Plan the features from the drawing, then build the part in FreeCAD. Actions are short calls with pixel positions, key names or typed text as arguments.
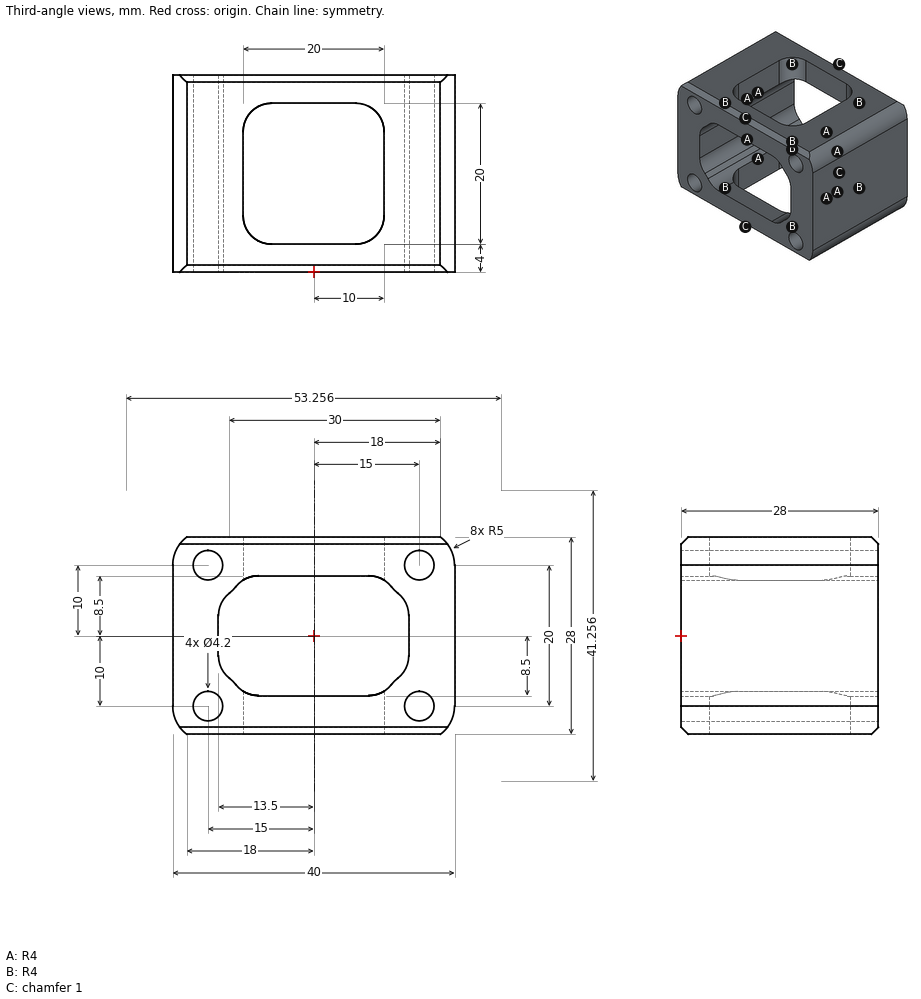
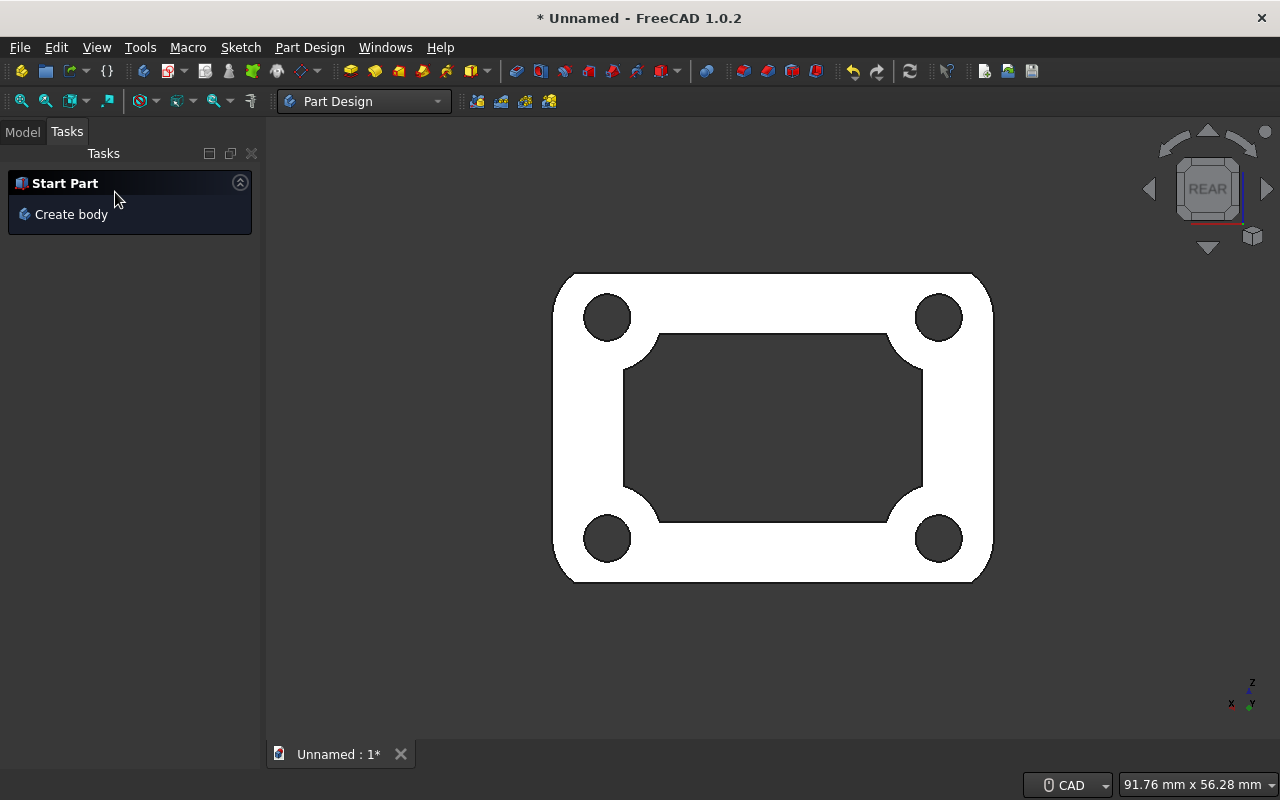
key(0)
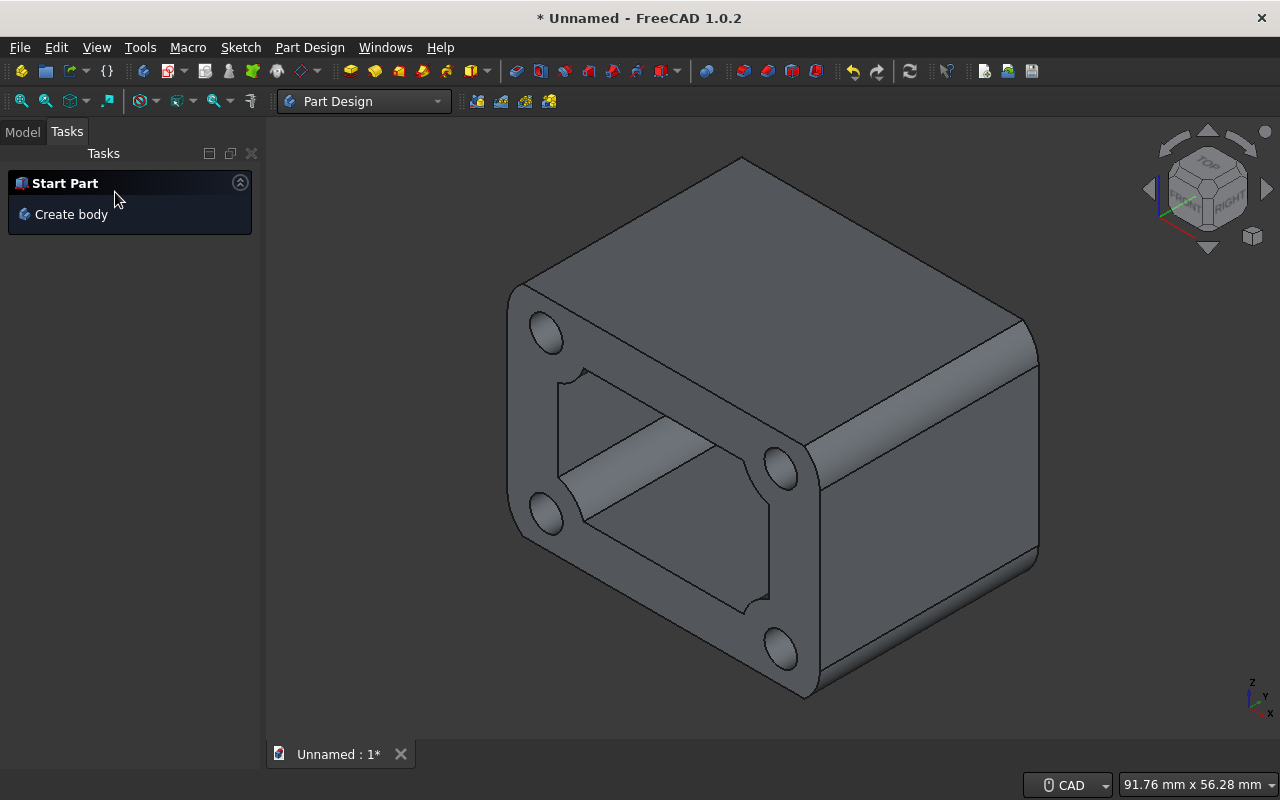
key(2)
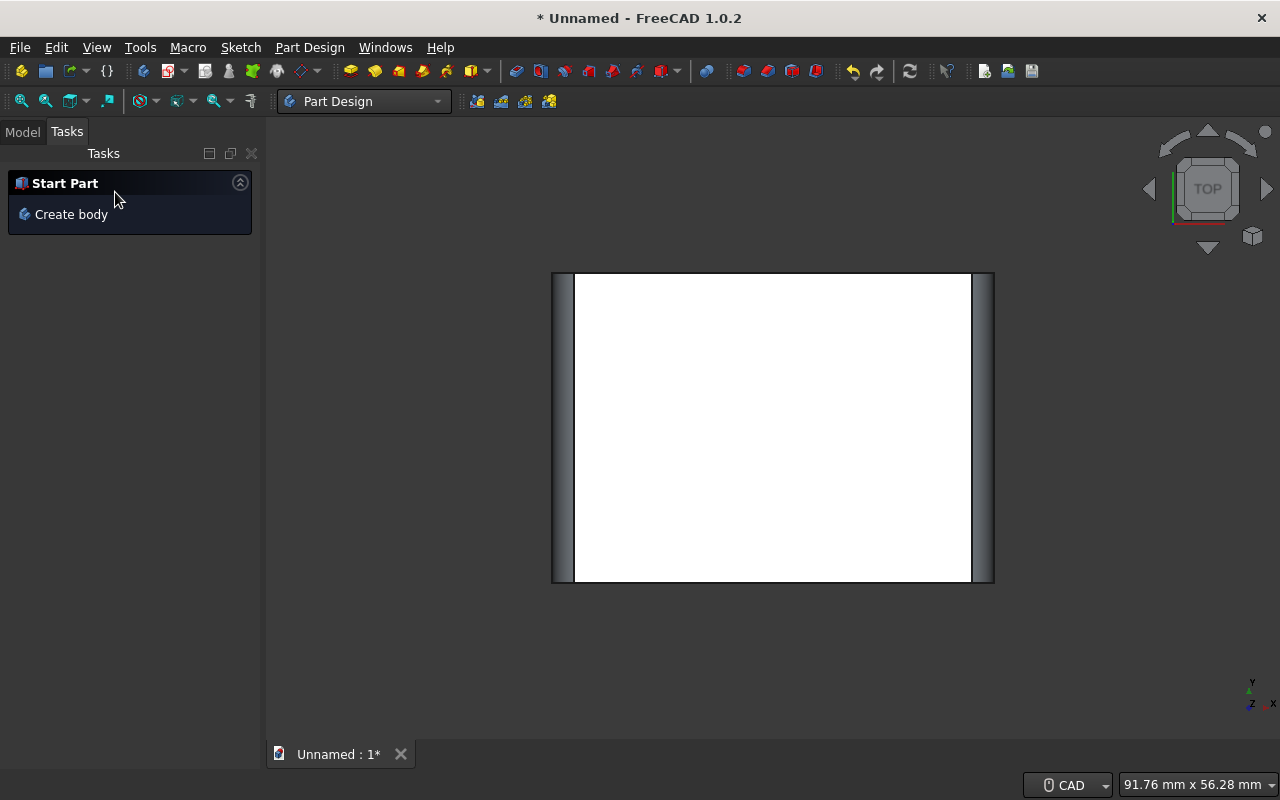
key(1)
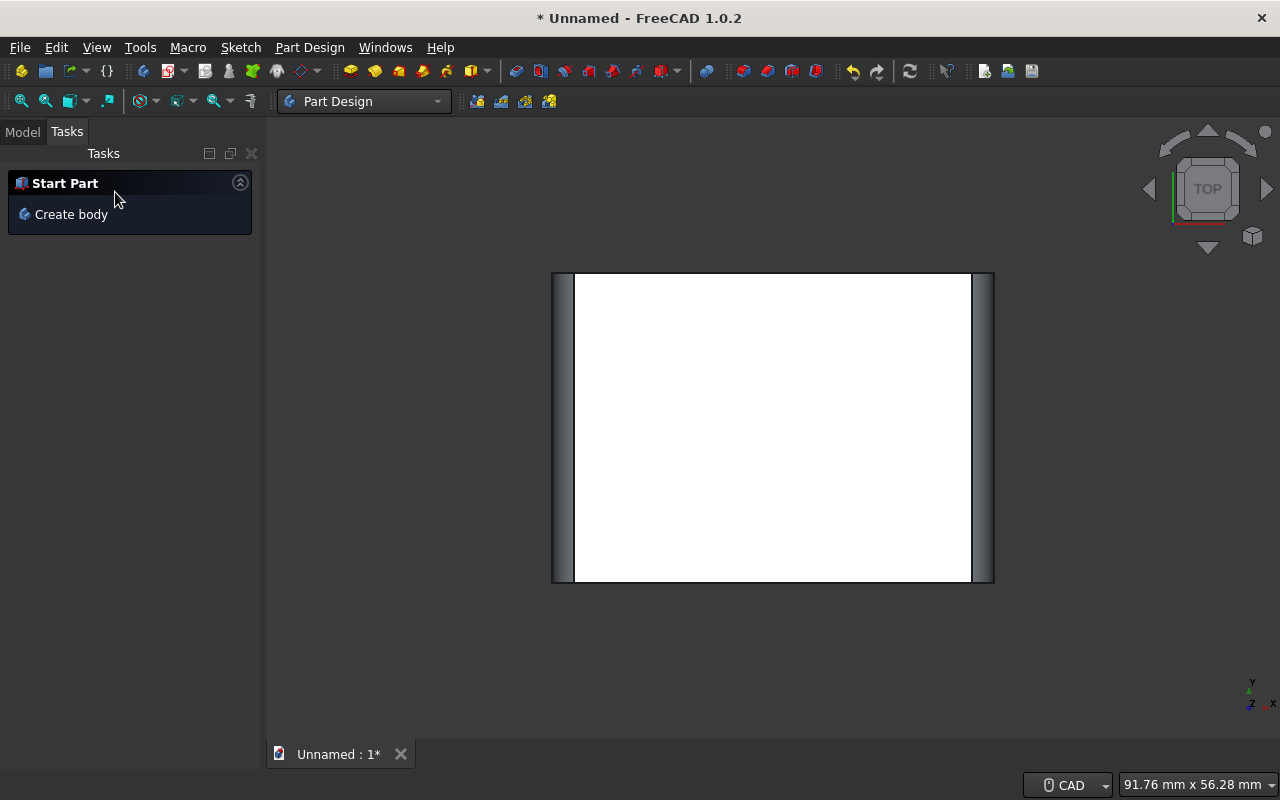
key(3)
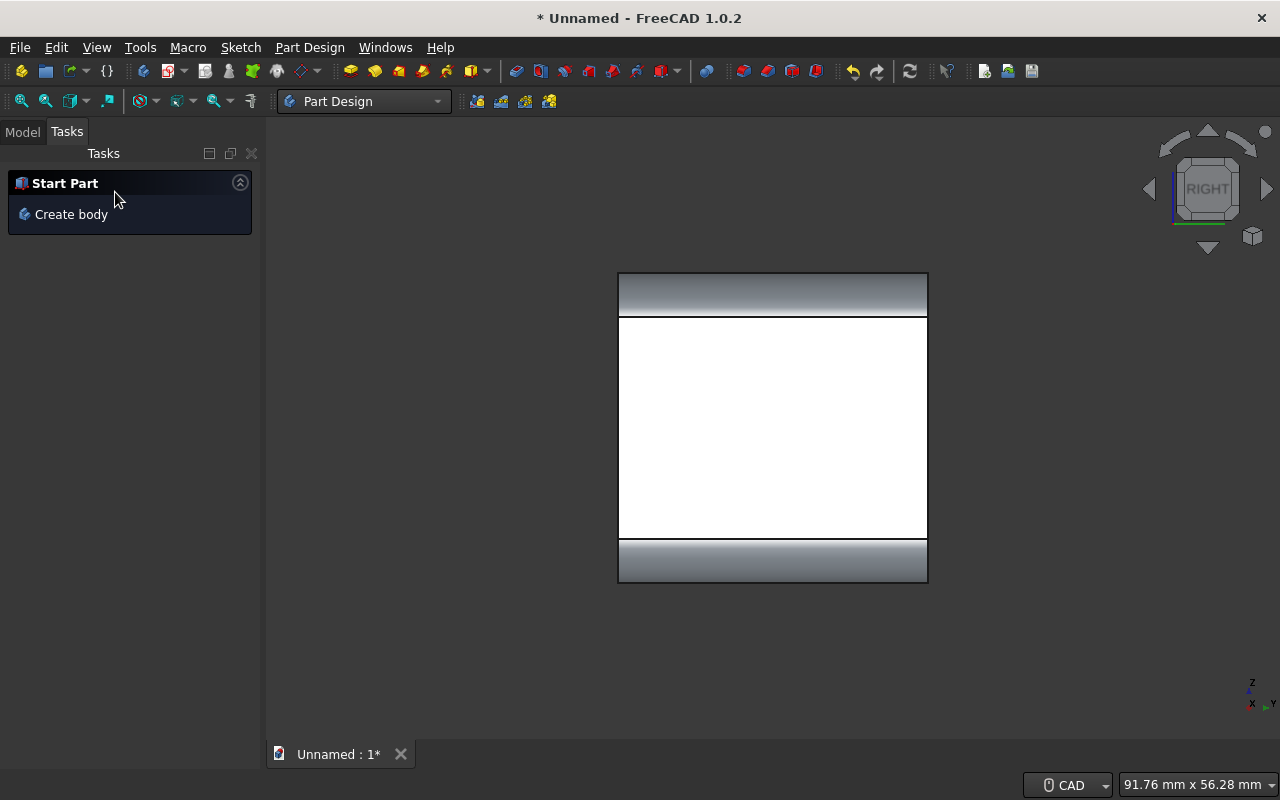
key(5)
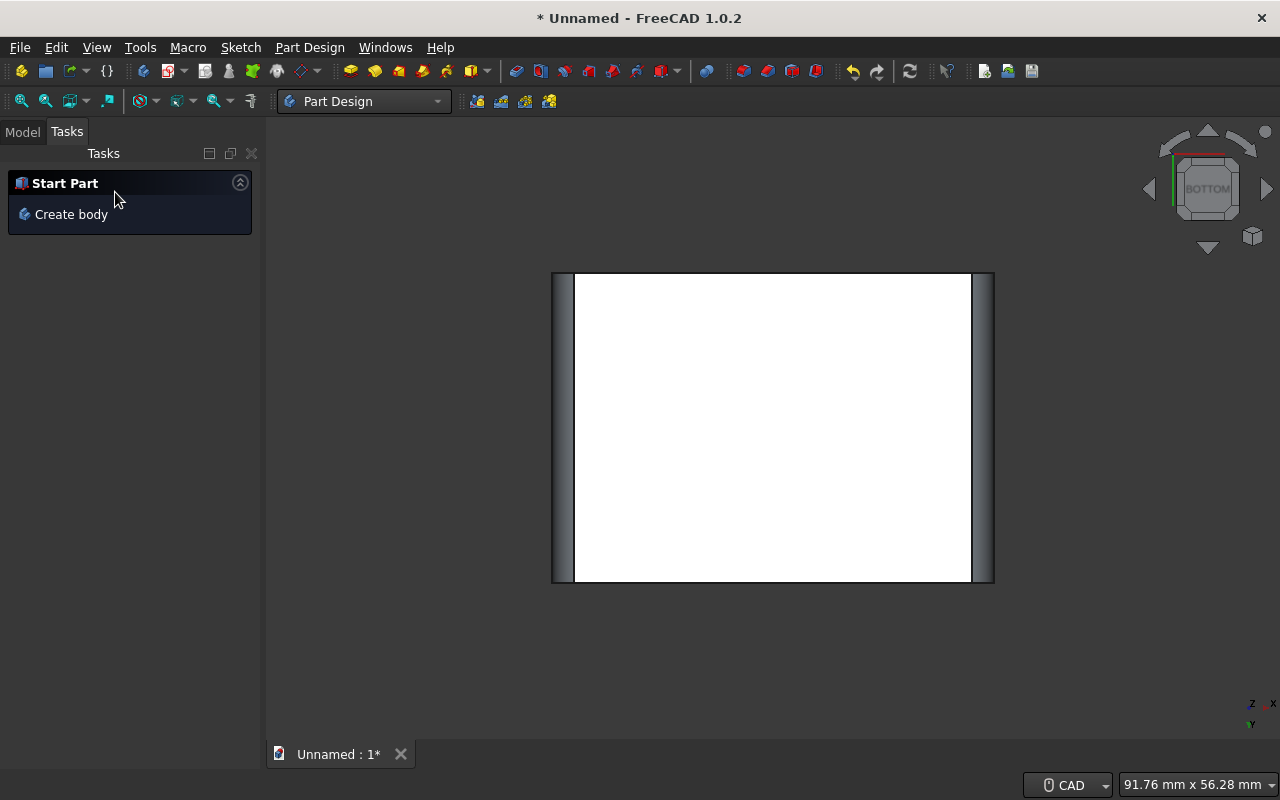
key(4)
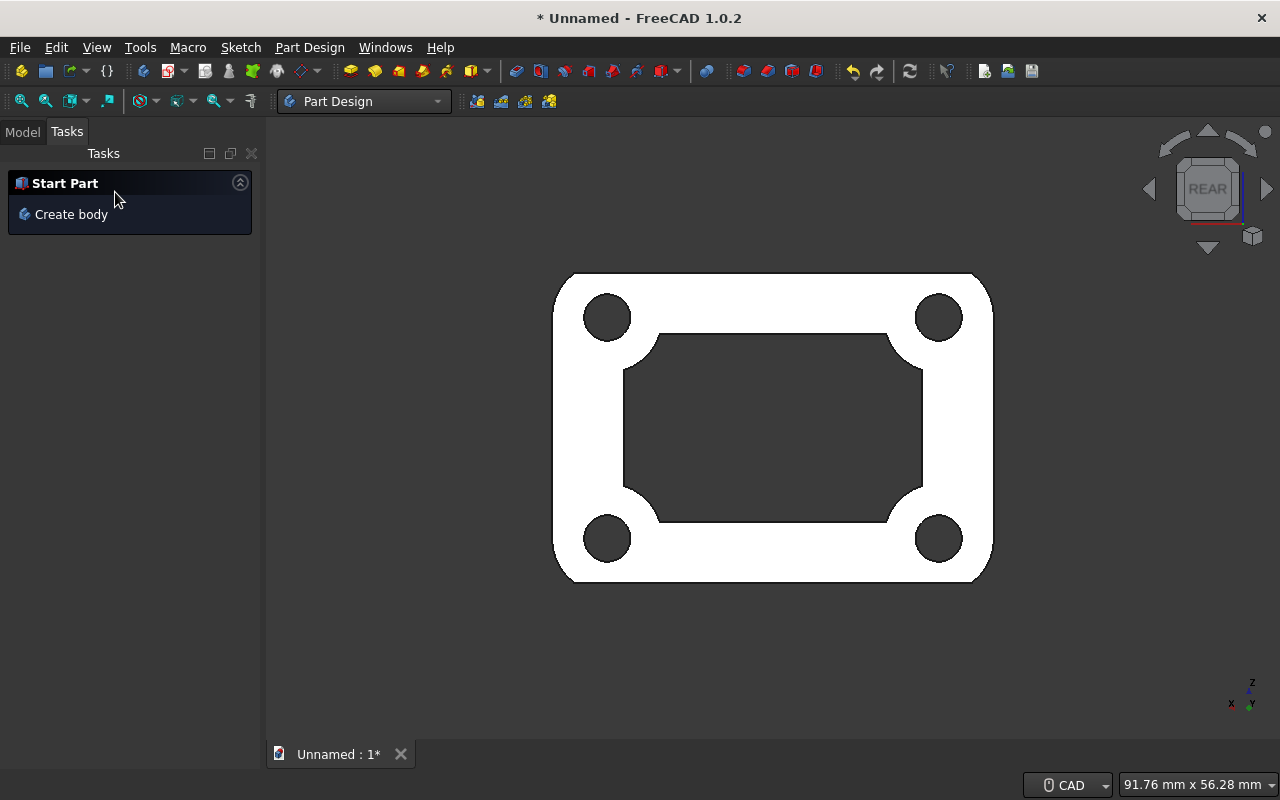
key(6)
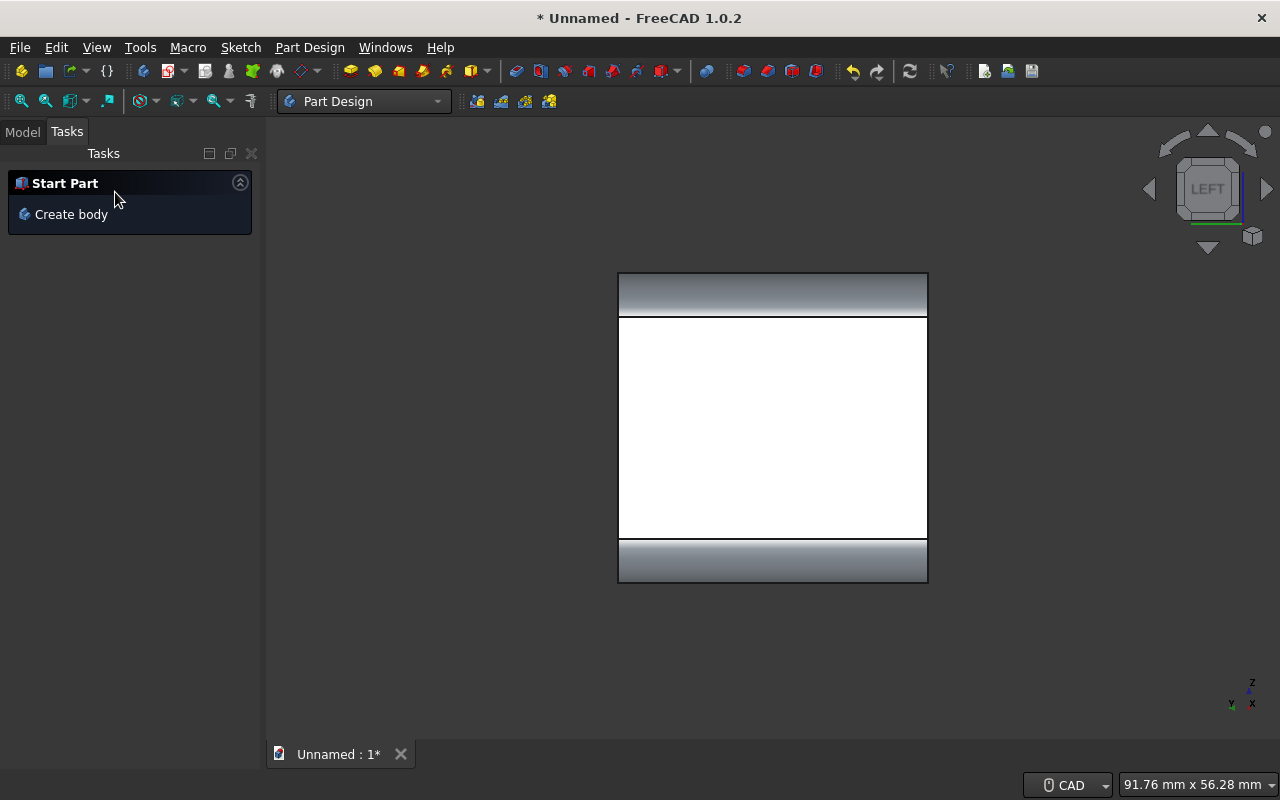
key(v)
key(3)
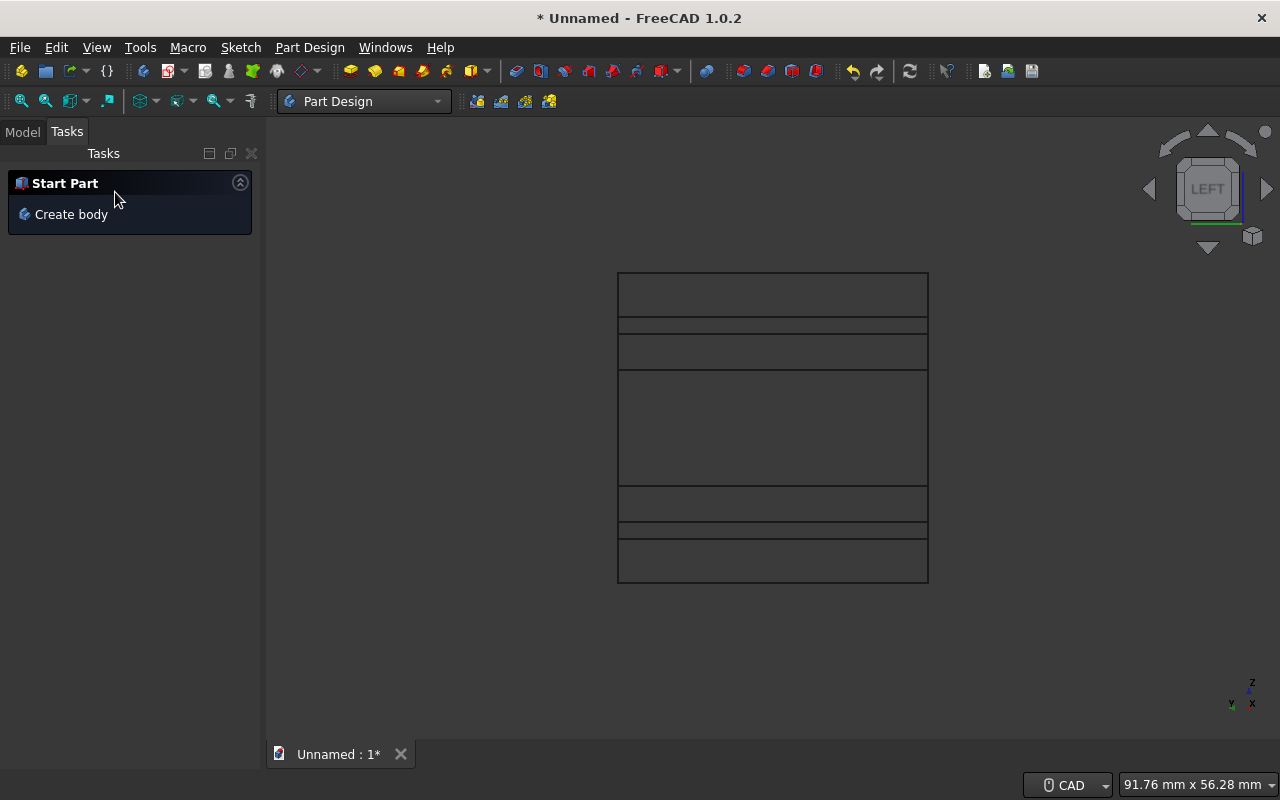
key(0)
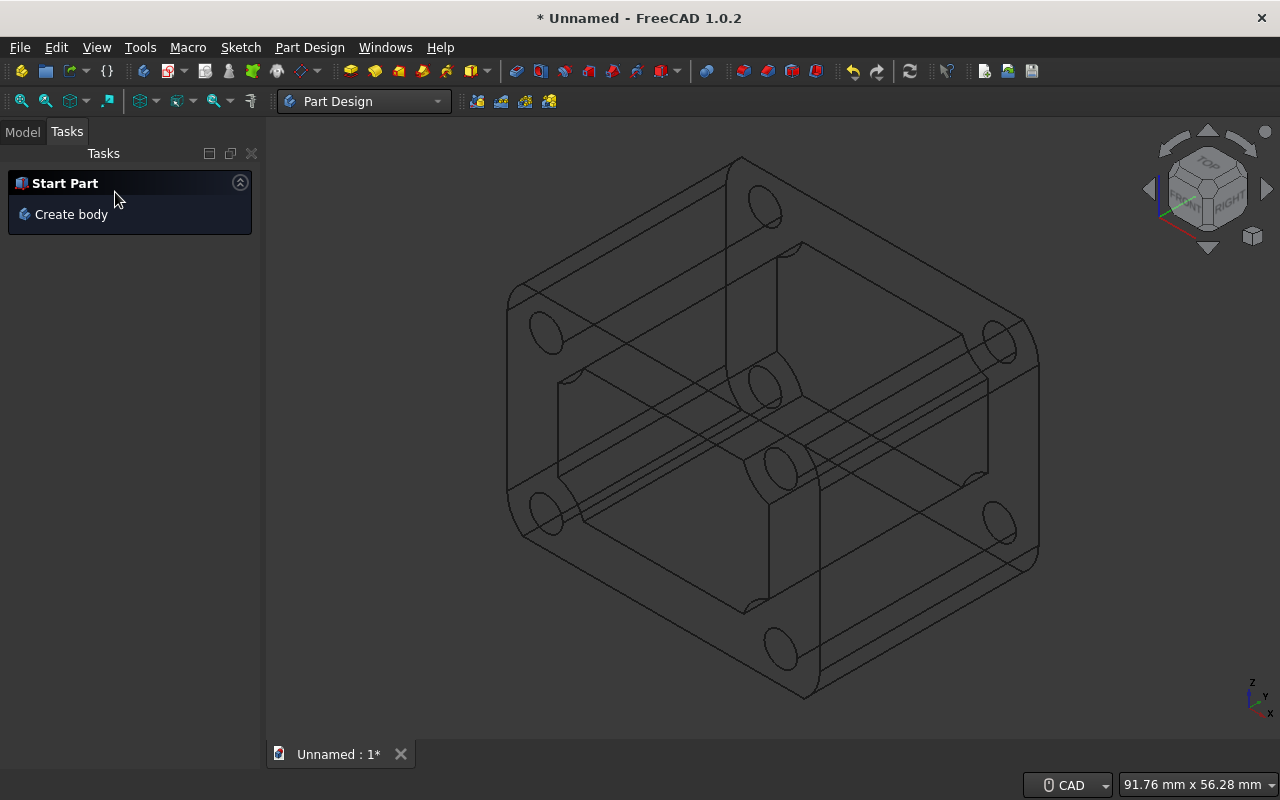
click(689, 401)